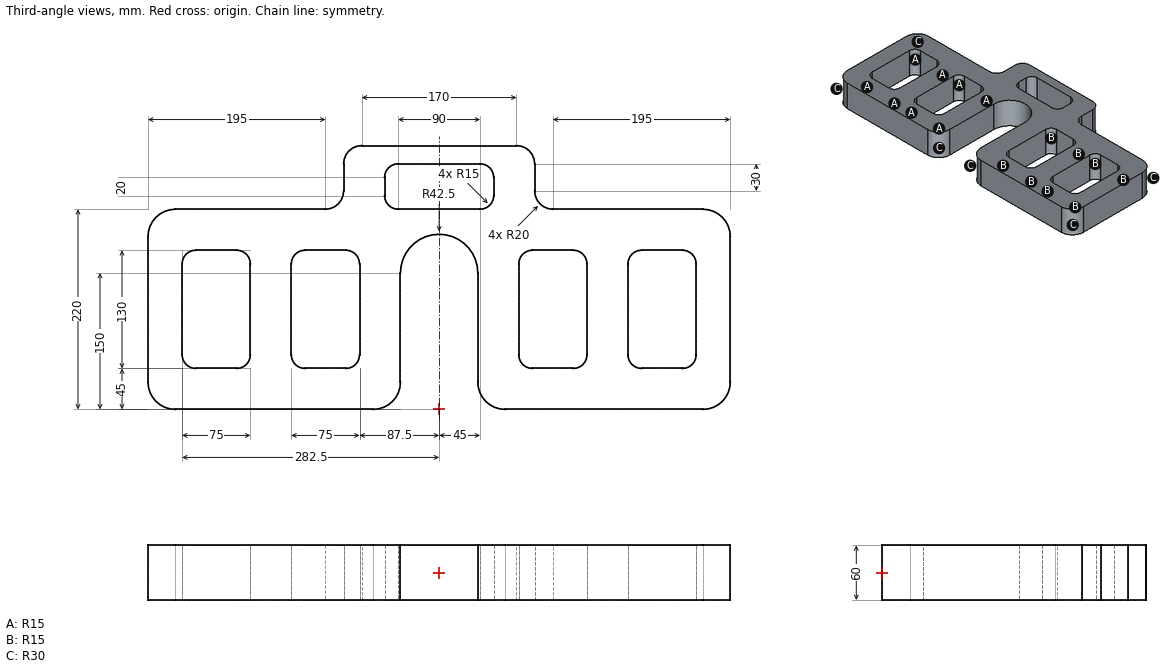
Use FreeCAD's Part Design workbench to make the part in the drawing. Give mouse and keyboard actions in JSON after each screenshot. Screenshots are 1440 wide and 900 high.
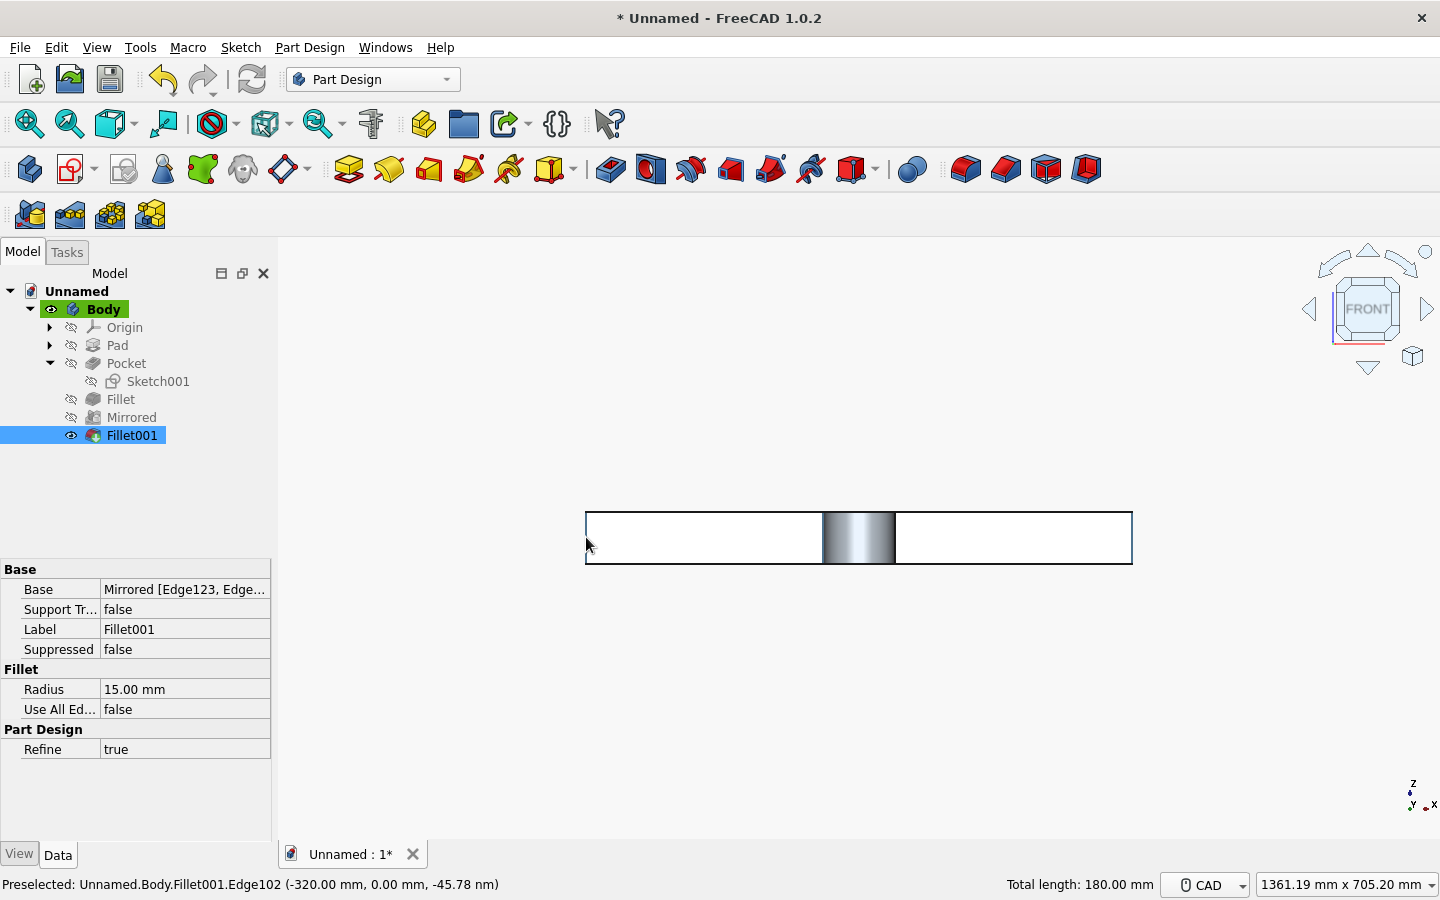
{"action": "left_click", "coordinate": [895, 537], "text": "ctrl"}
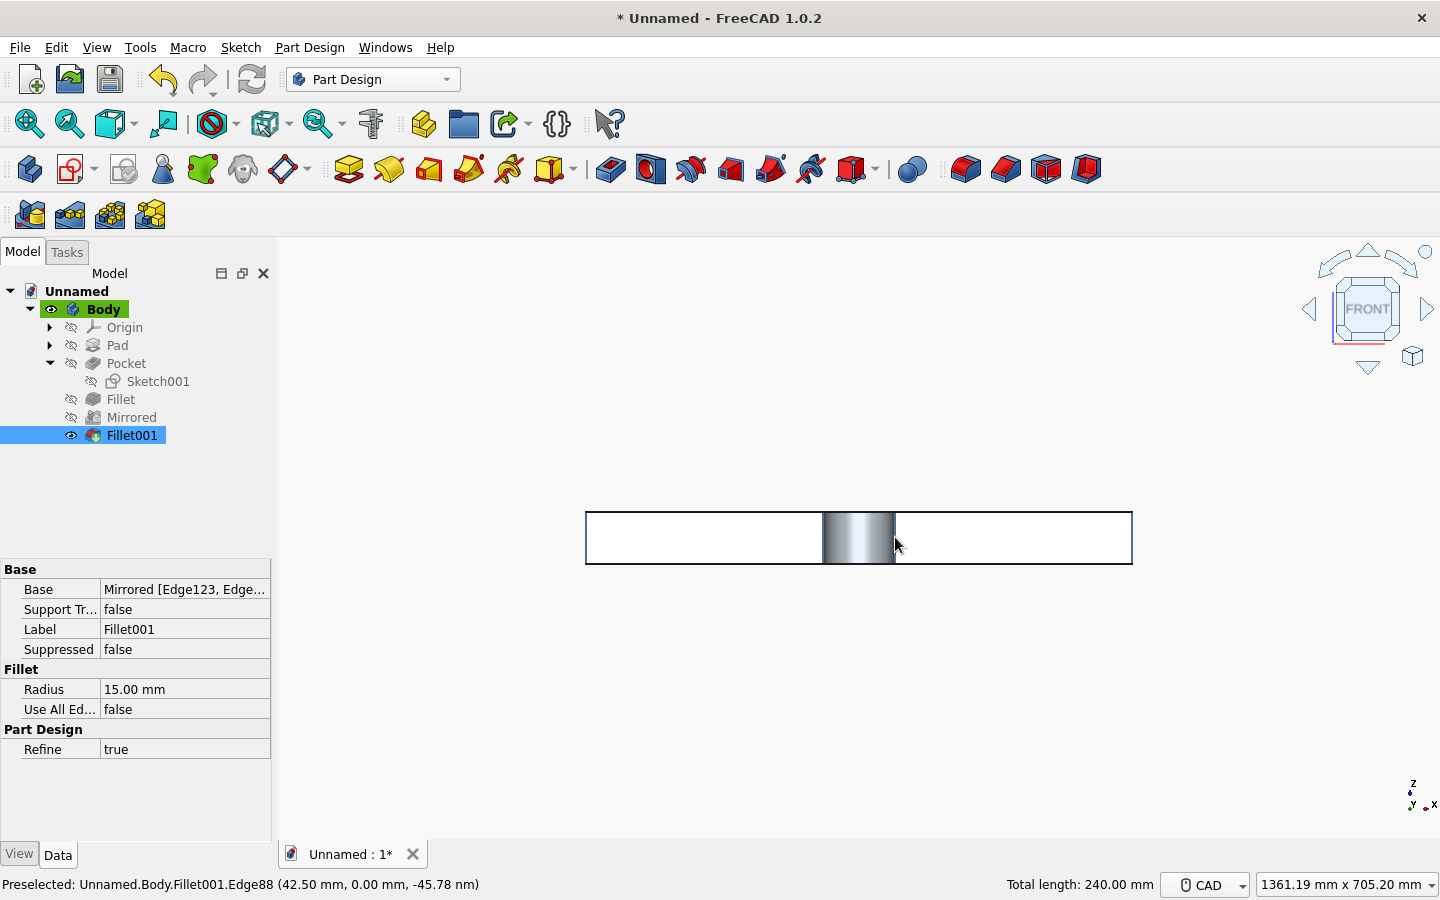
{"action": "key", "text": "3"}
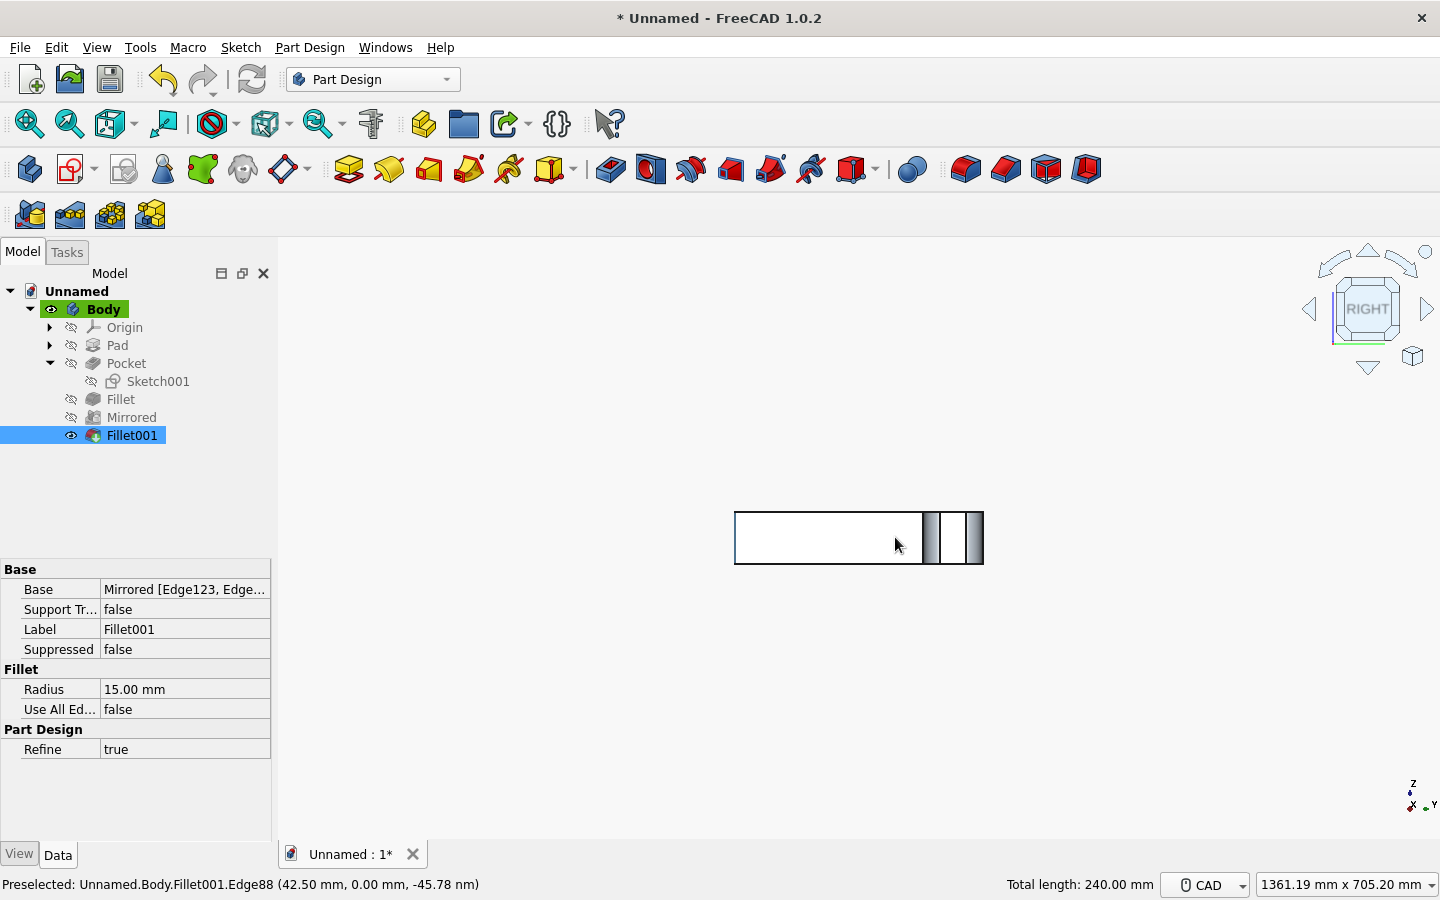
{"action": "left_click", "coordinate": [30, 124]}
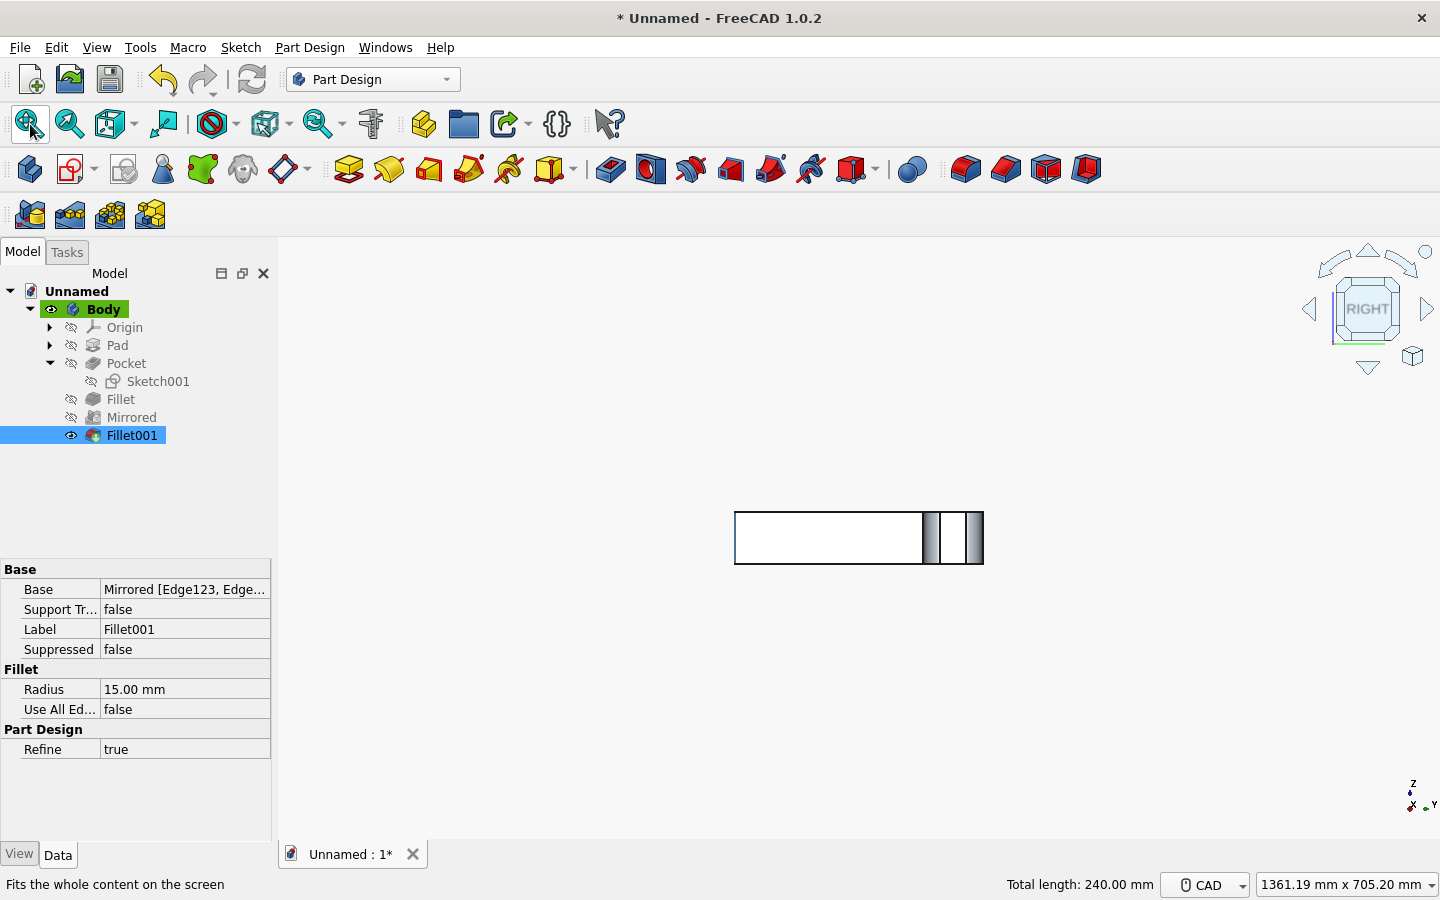
{"action": "left_click", "coordinate": [923, 537], "text": "ctrl"}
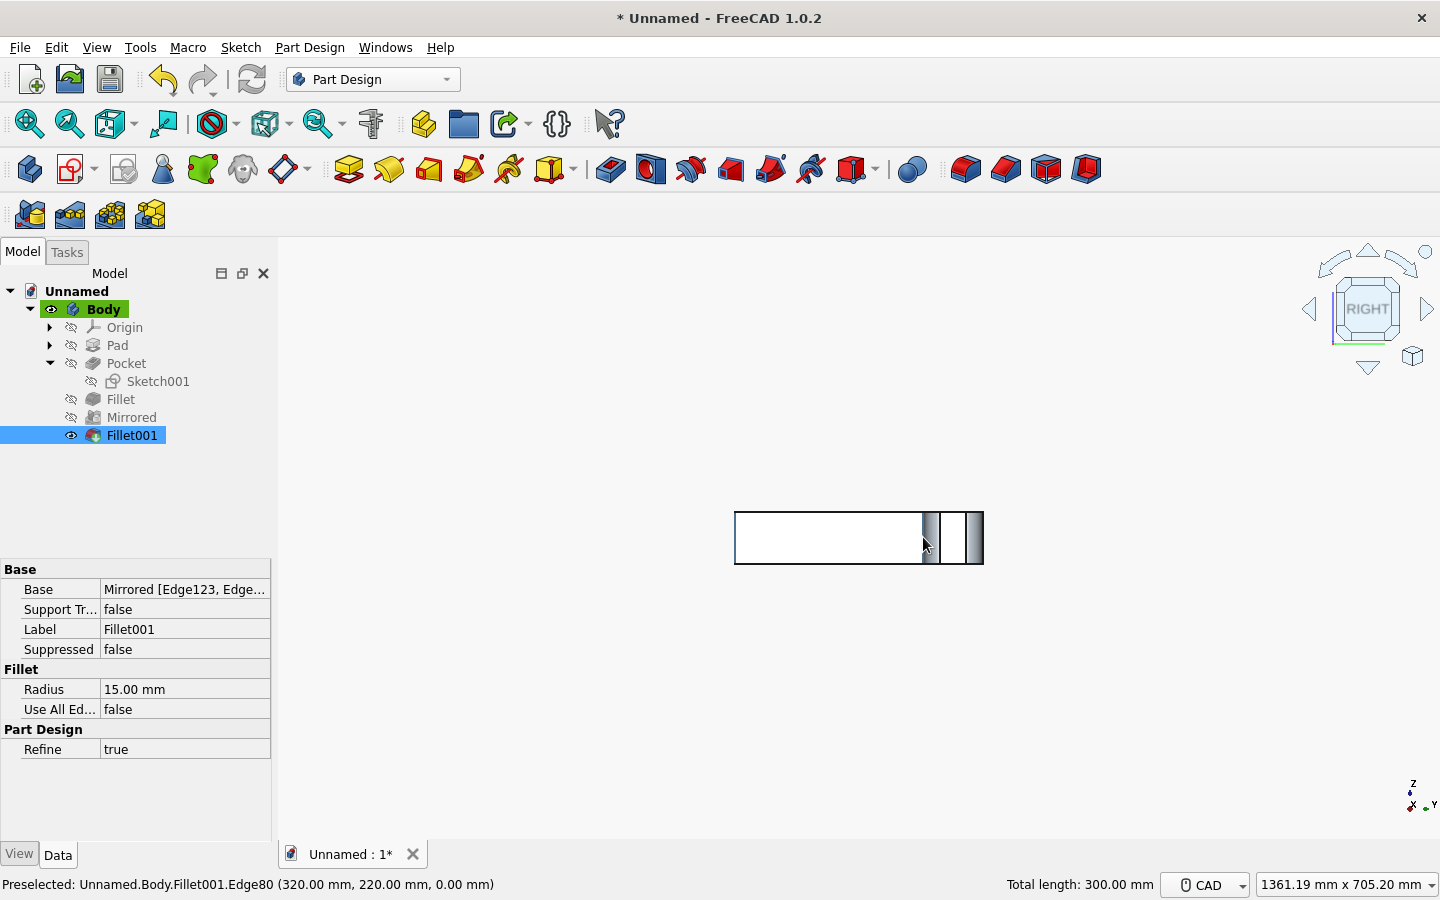
{"action": "key", "text": "5"}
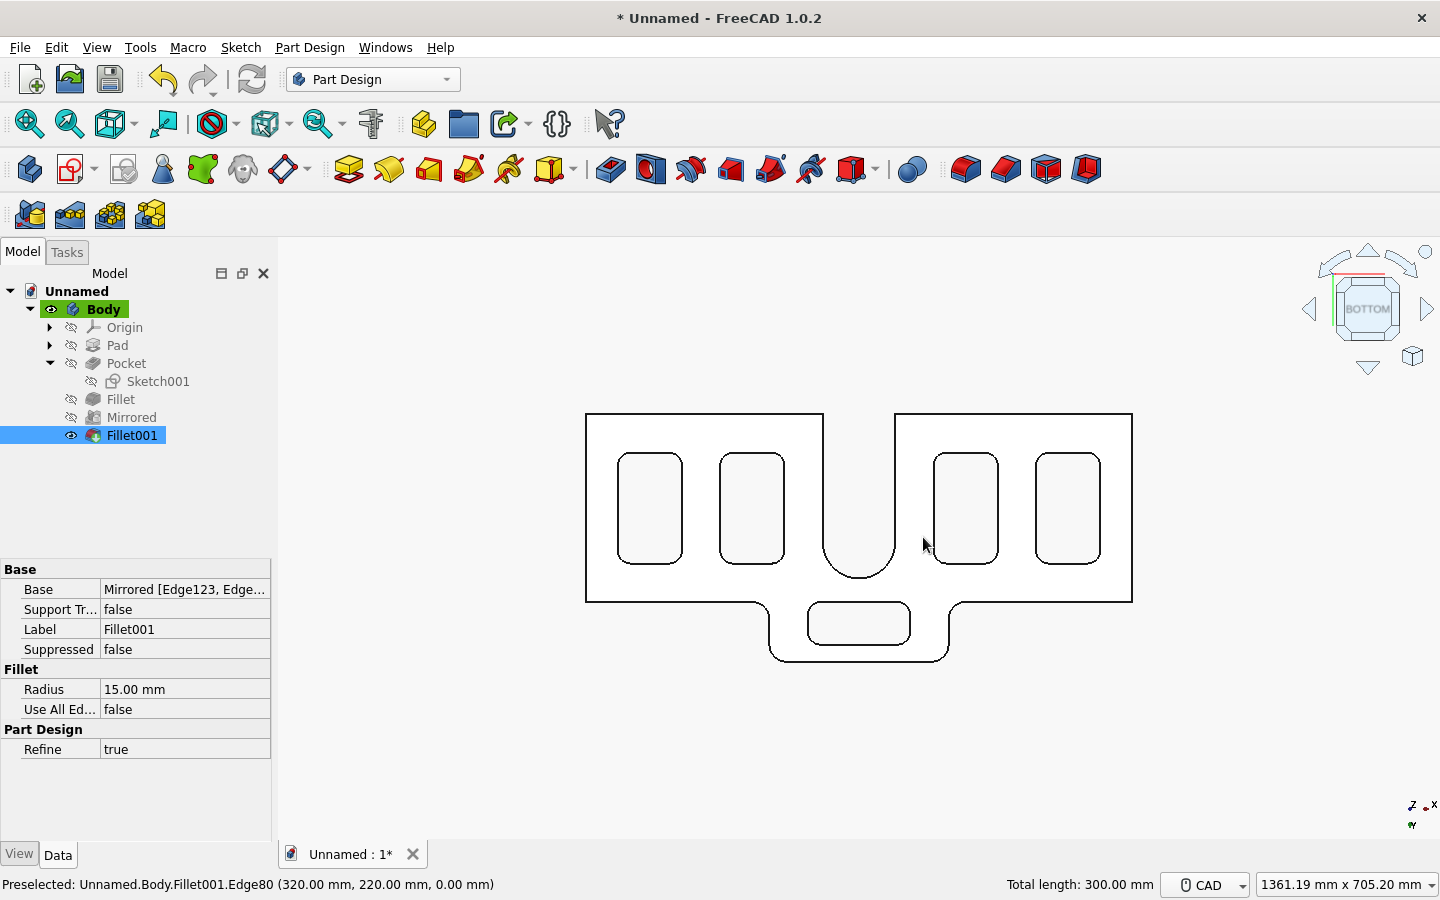
{"action": "key", "text": "4"}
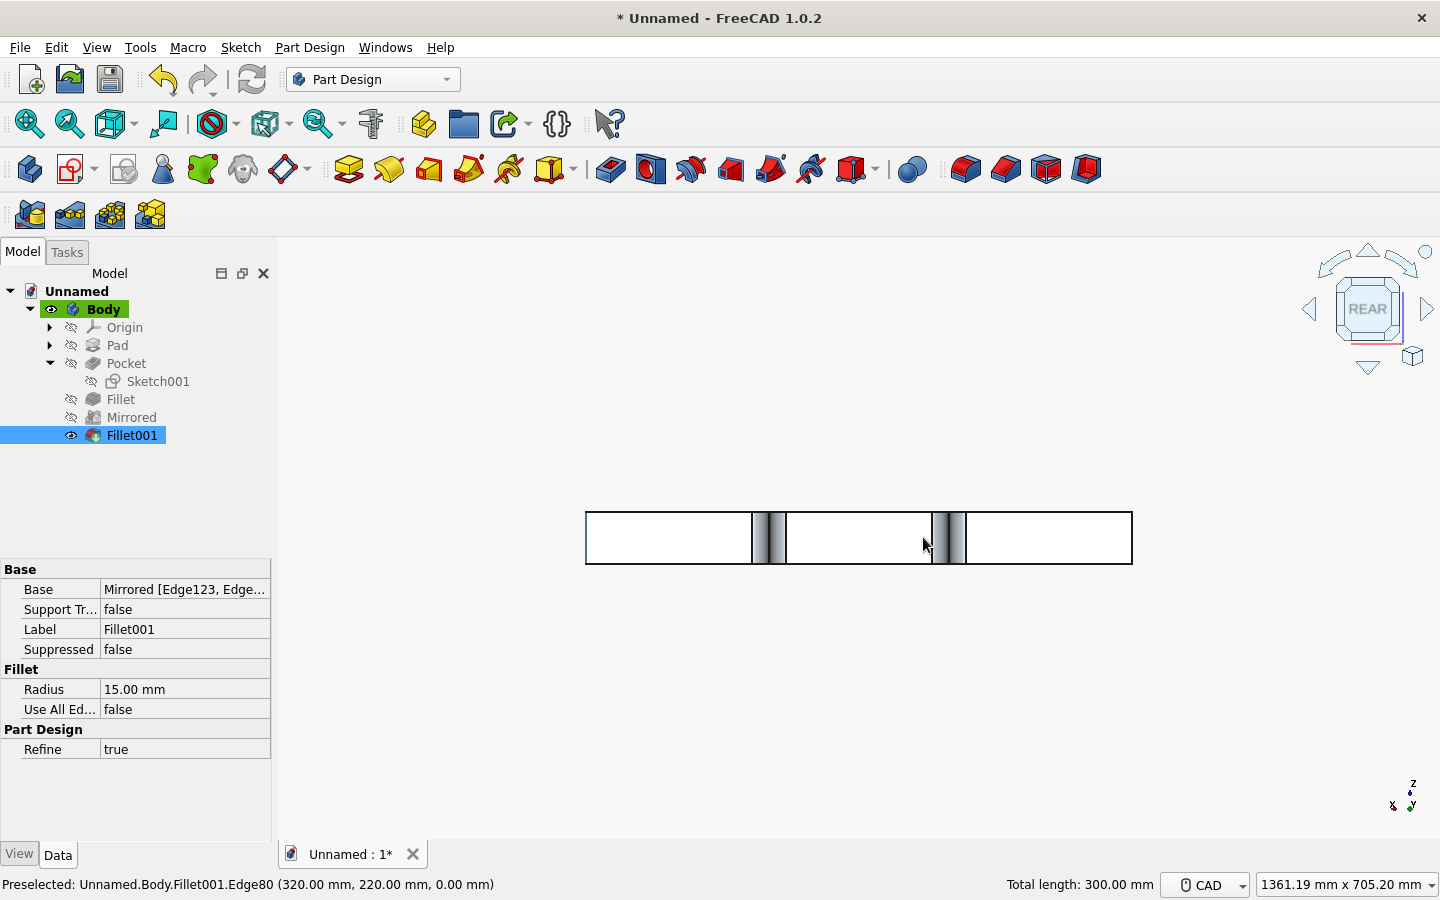
{"action": "left_click", "coordinate": [1132, 537], "text": "ctrl"}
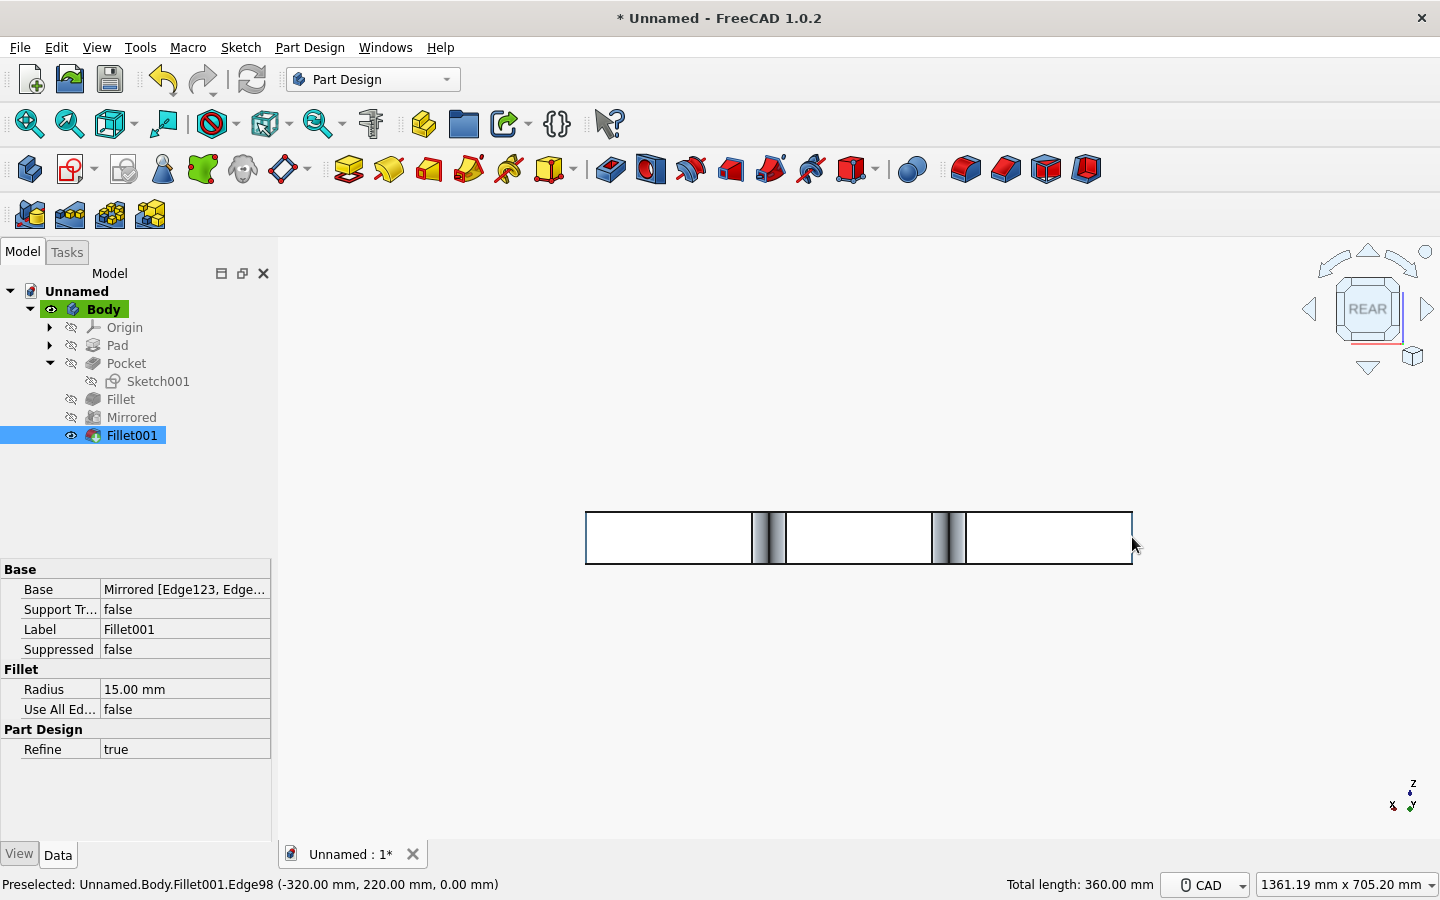
{"action": "left_click", "coordinate": [966, 170]}